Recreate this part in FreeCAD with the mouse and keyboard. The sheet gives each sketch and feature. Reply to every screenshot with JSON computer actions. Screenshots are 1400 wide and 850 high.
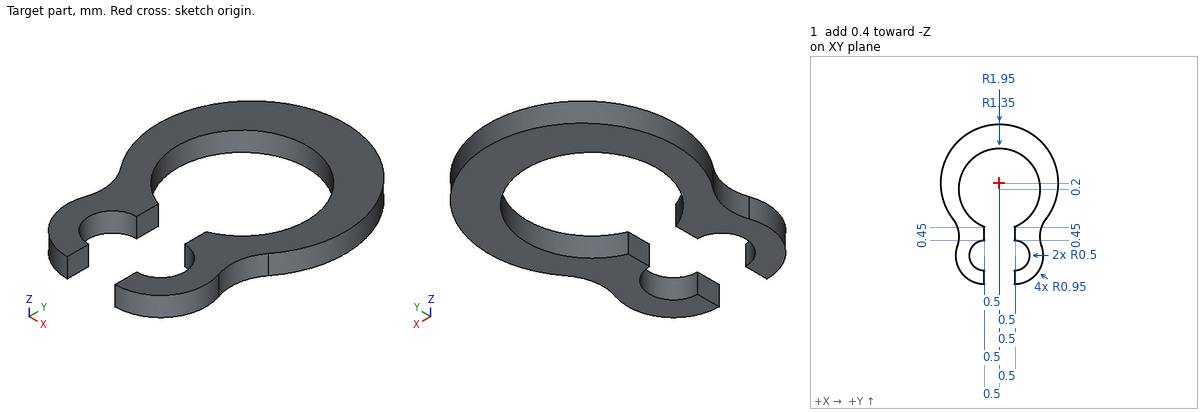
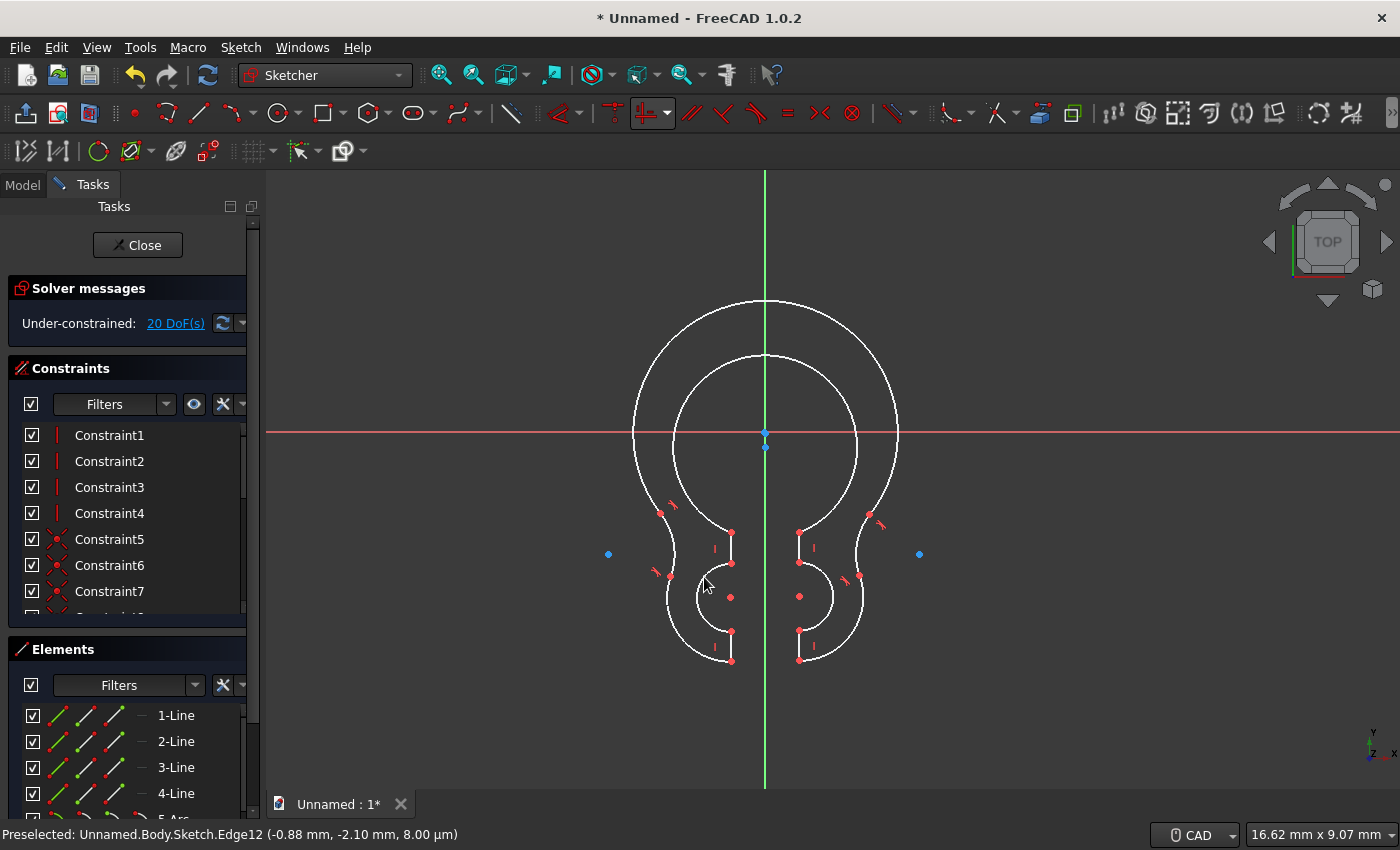
{"action": "left_click_drag", "start_coordinate": [755, 422], "coordinate": [776, 443]}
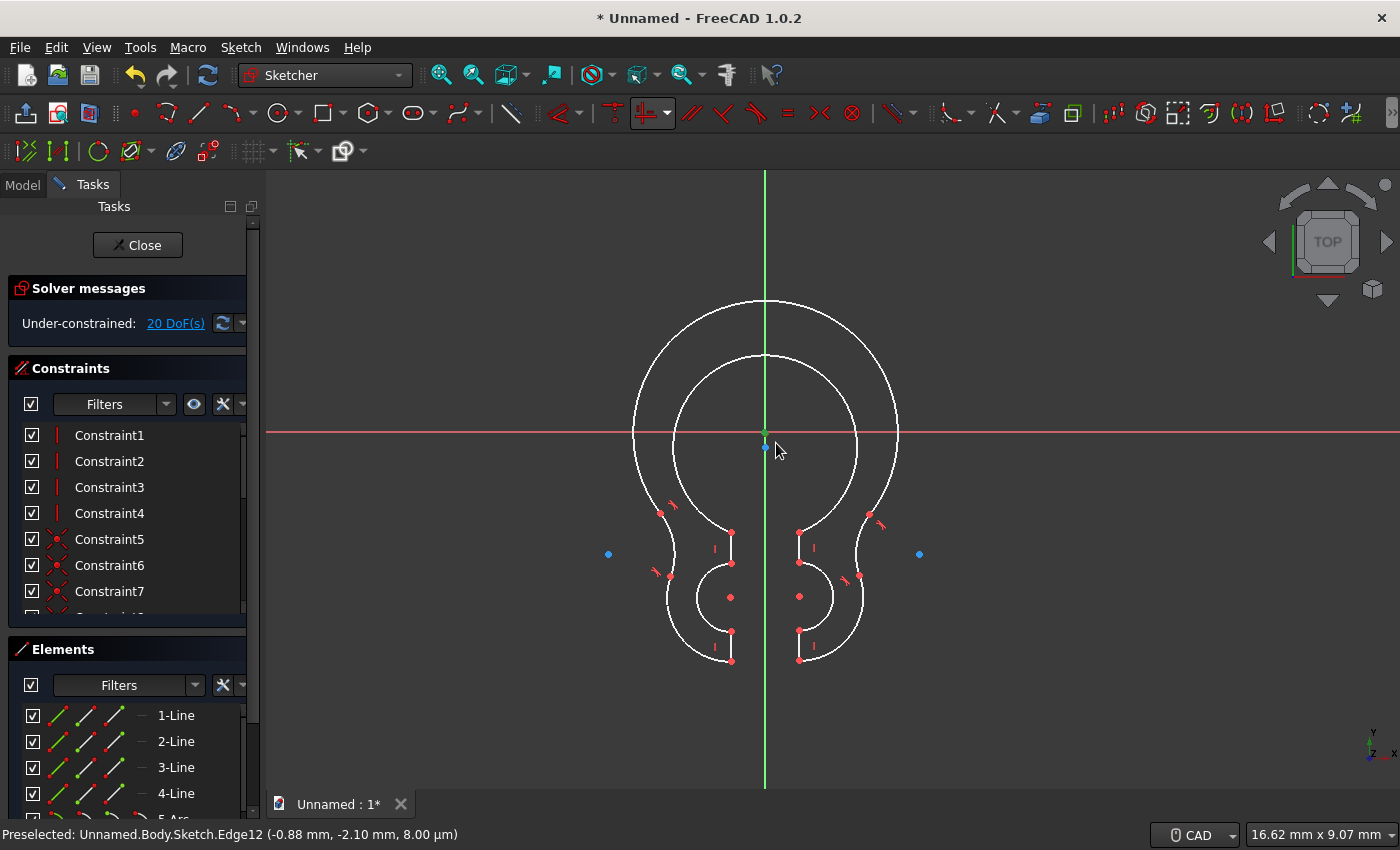
{"action": "key", "text": "c"}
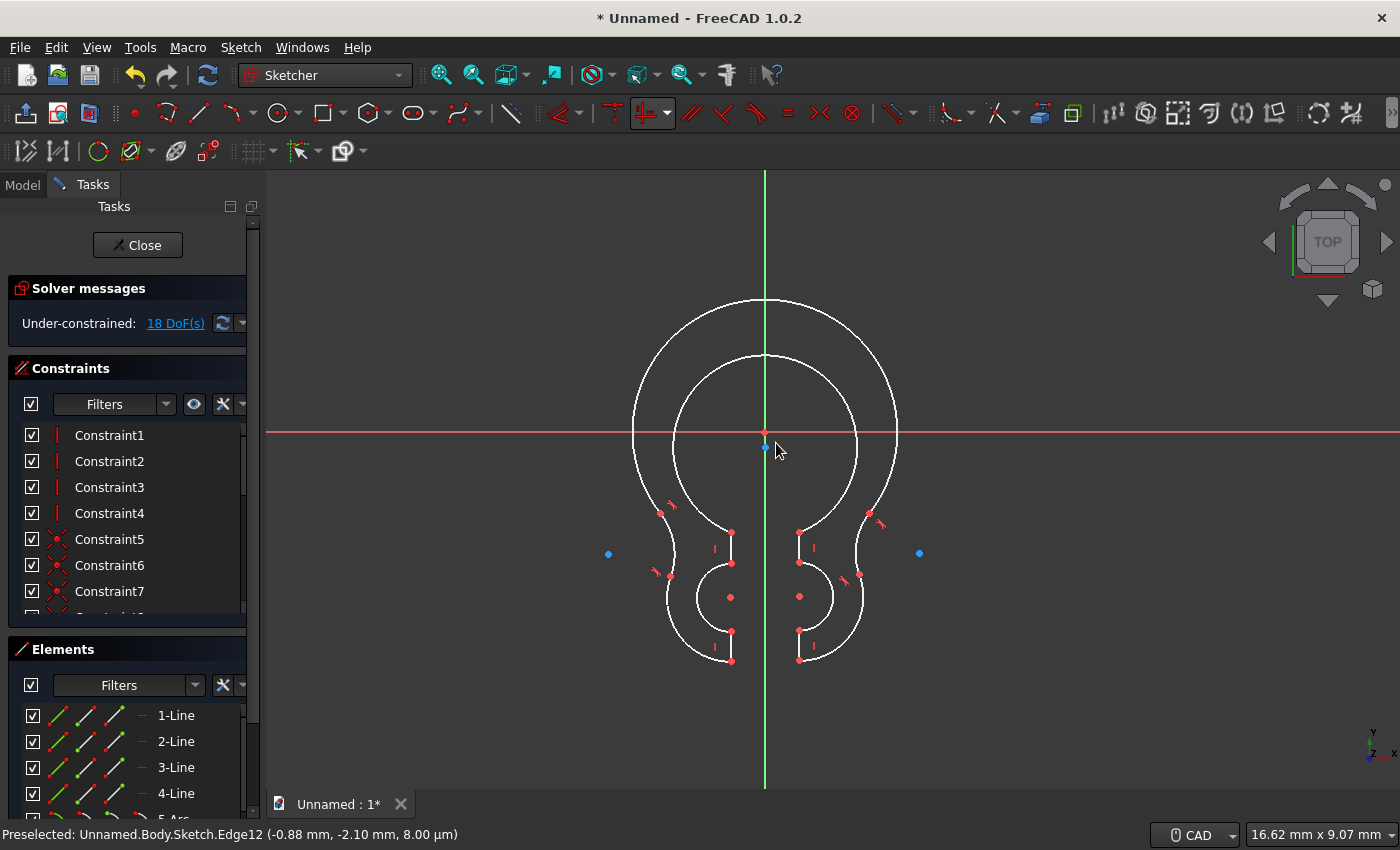
{"action": "left_click", "coordinate": [834, 651]}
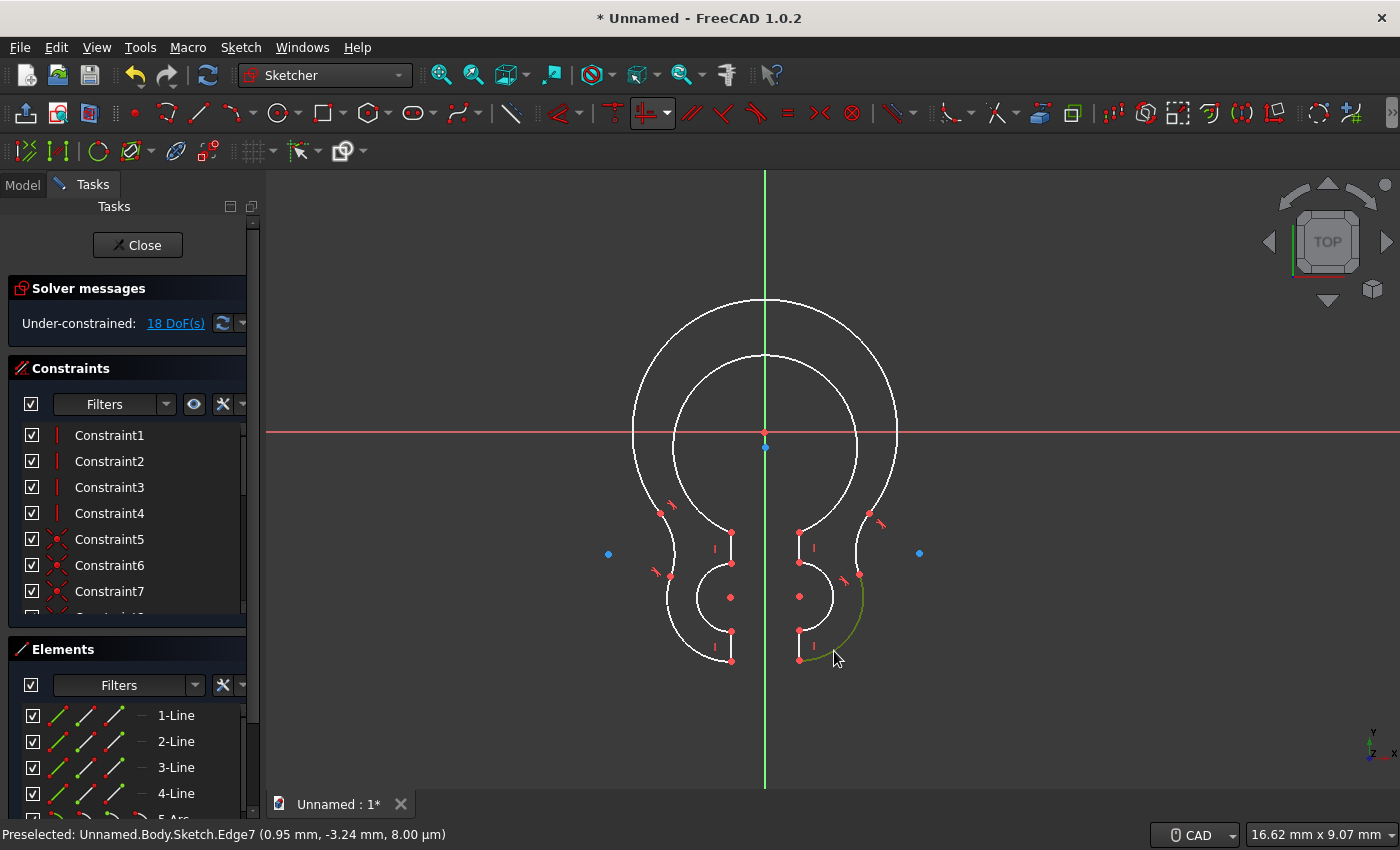
{"action": "left_click", "coordinate": [860, 531]}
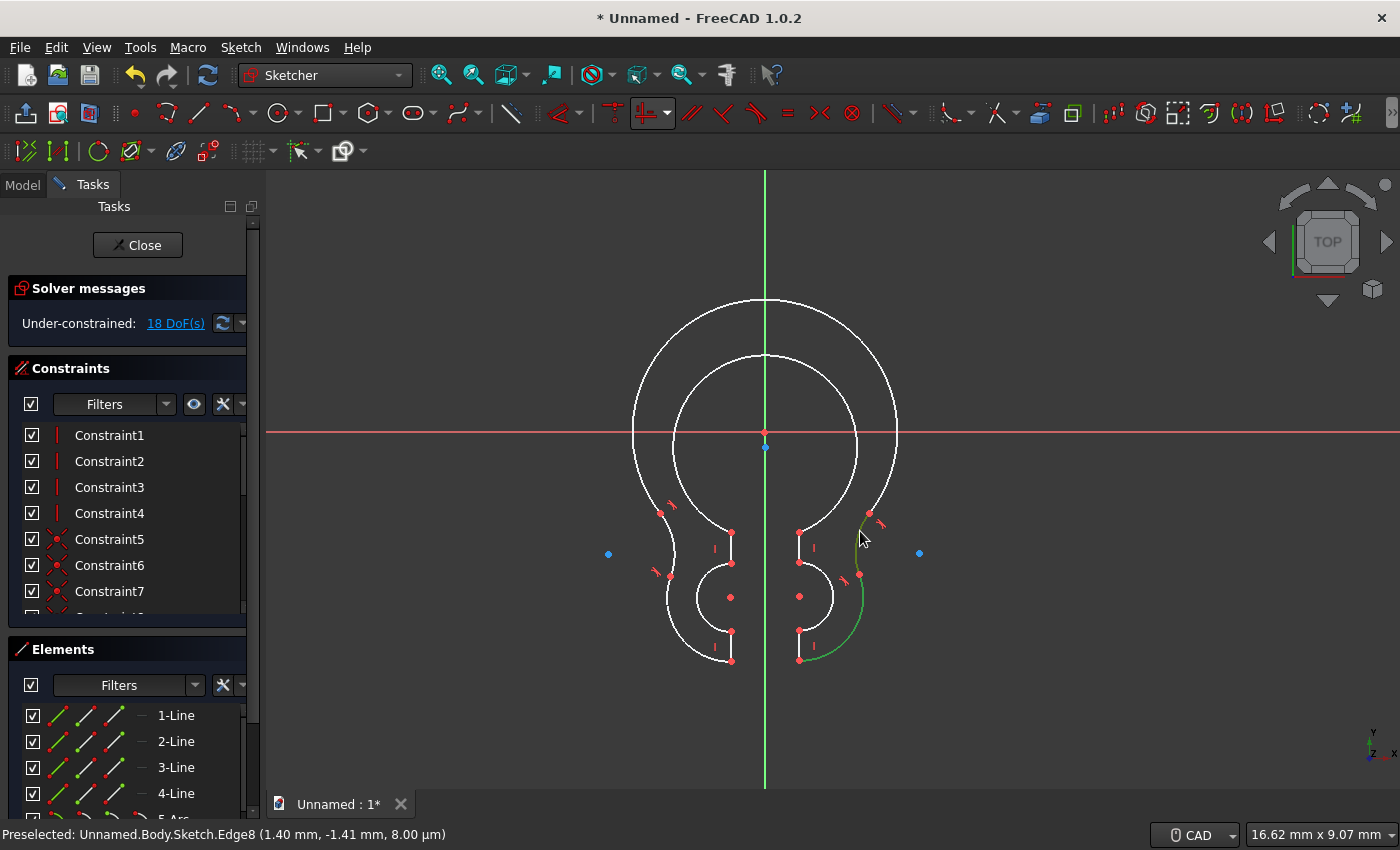
{"action": "left_click", "coordinate": [675, 557]}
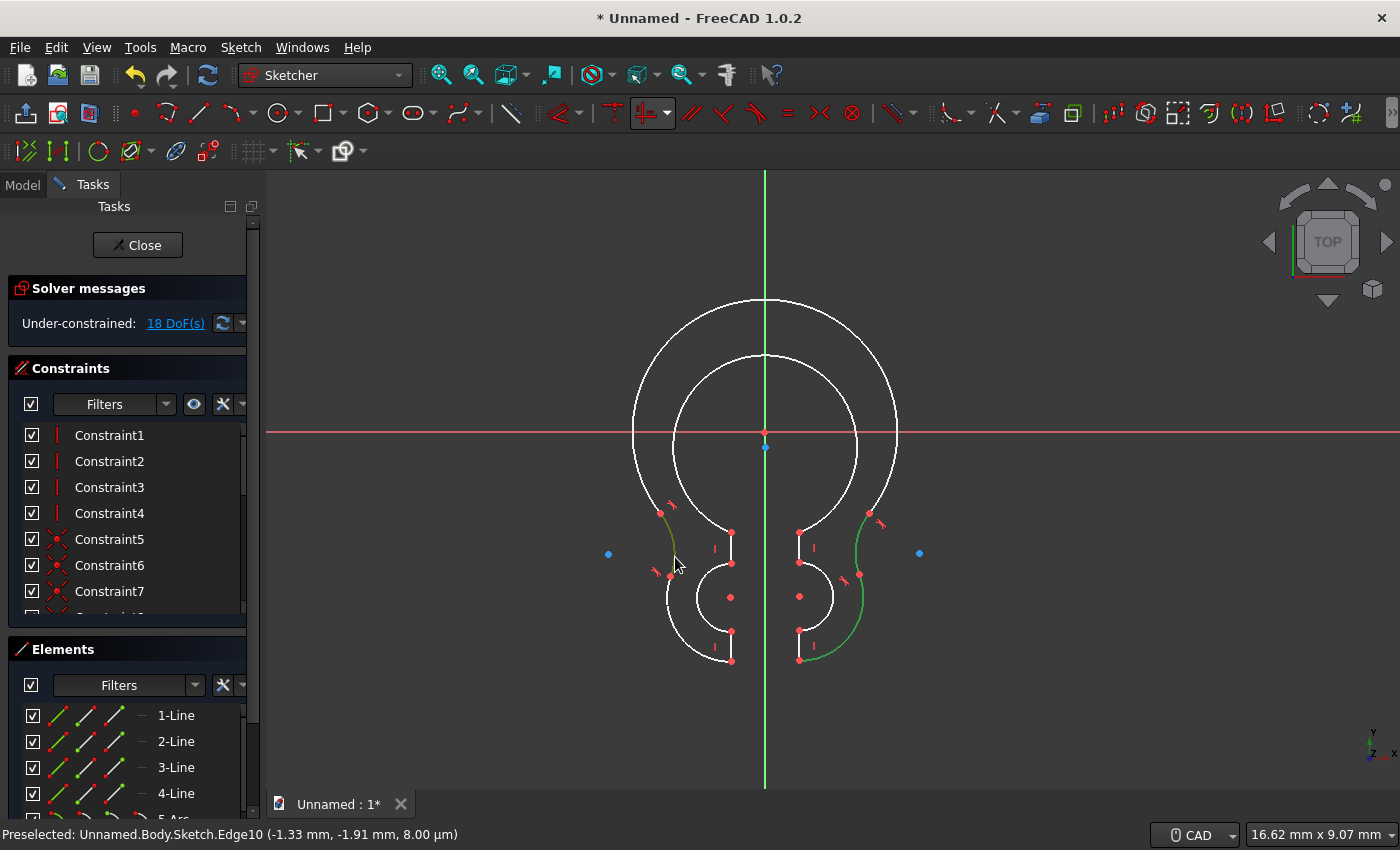
{"action": "left_click", "coordinate": [669, 613]}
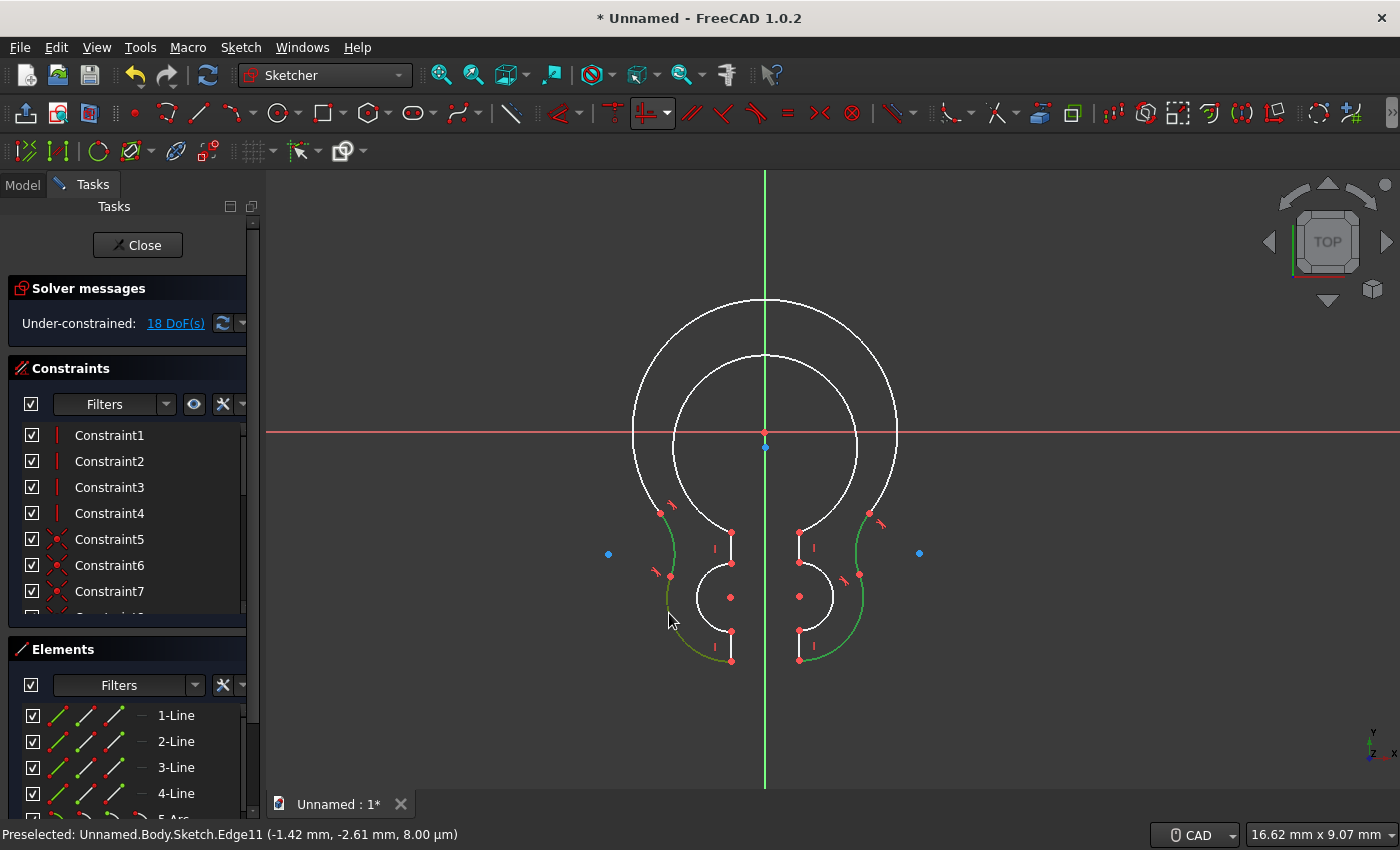
{"action": "left_click", "coordinate": [788, 114]}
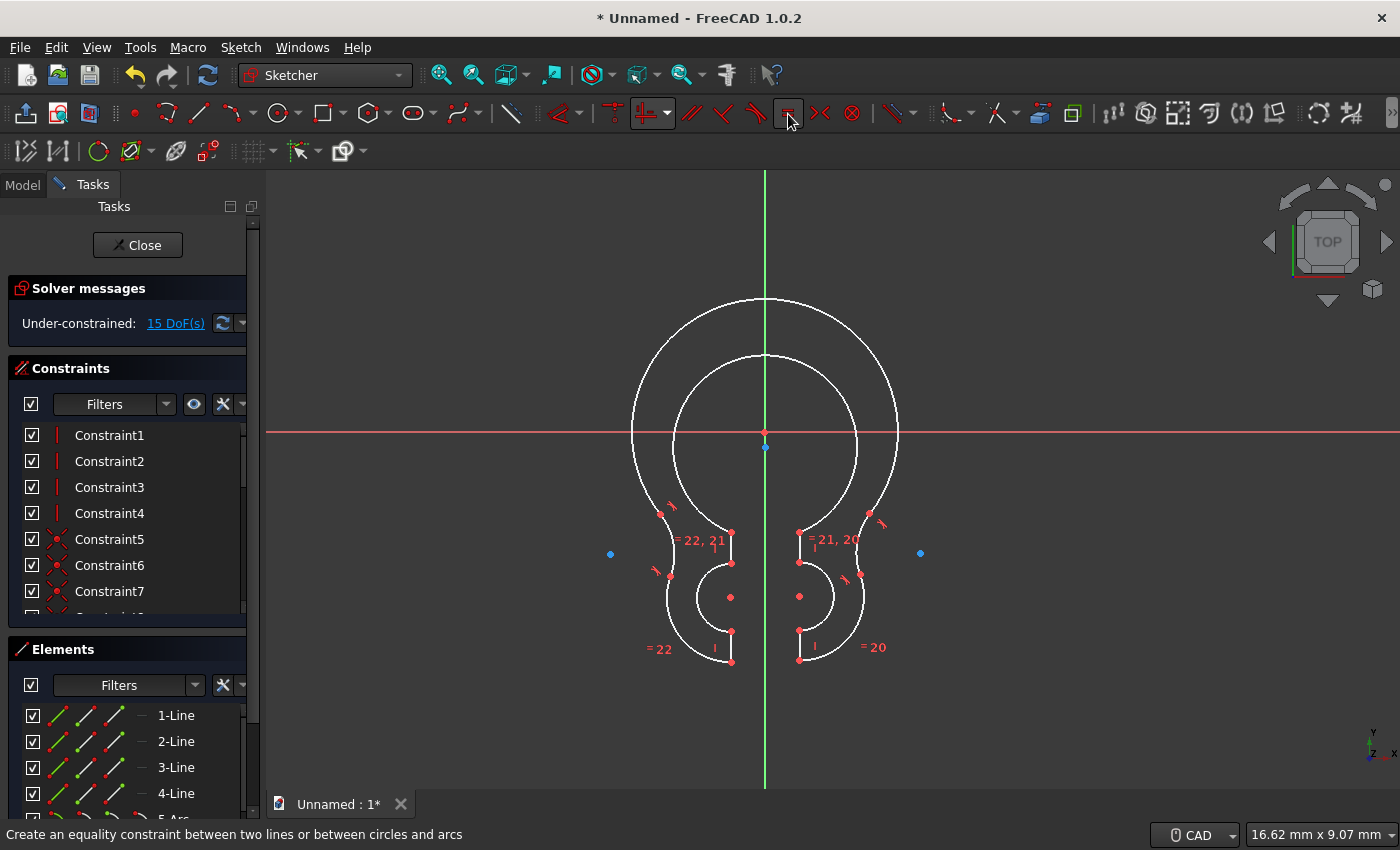
{"action": "left_click", "coordinate": [827, 616]}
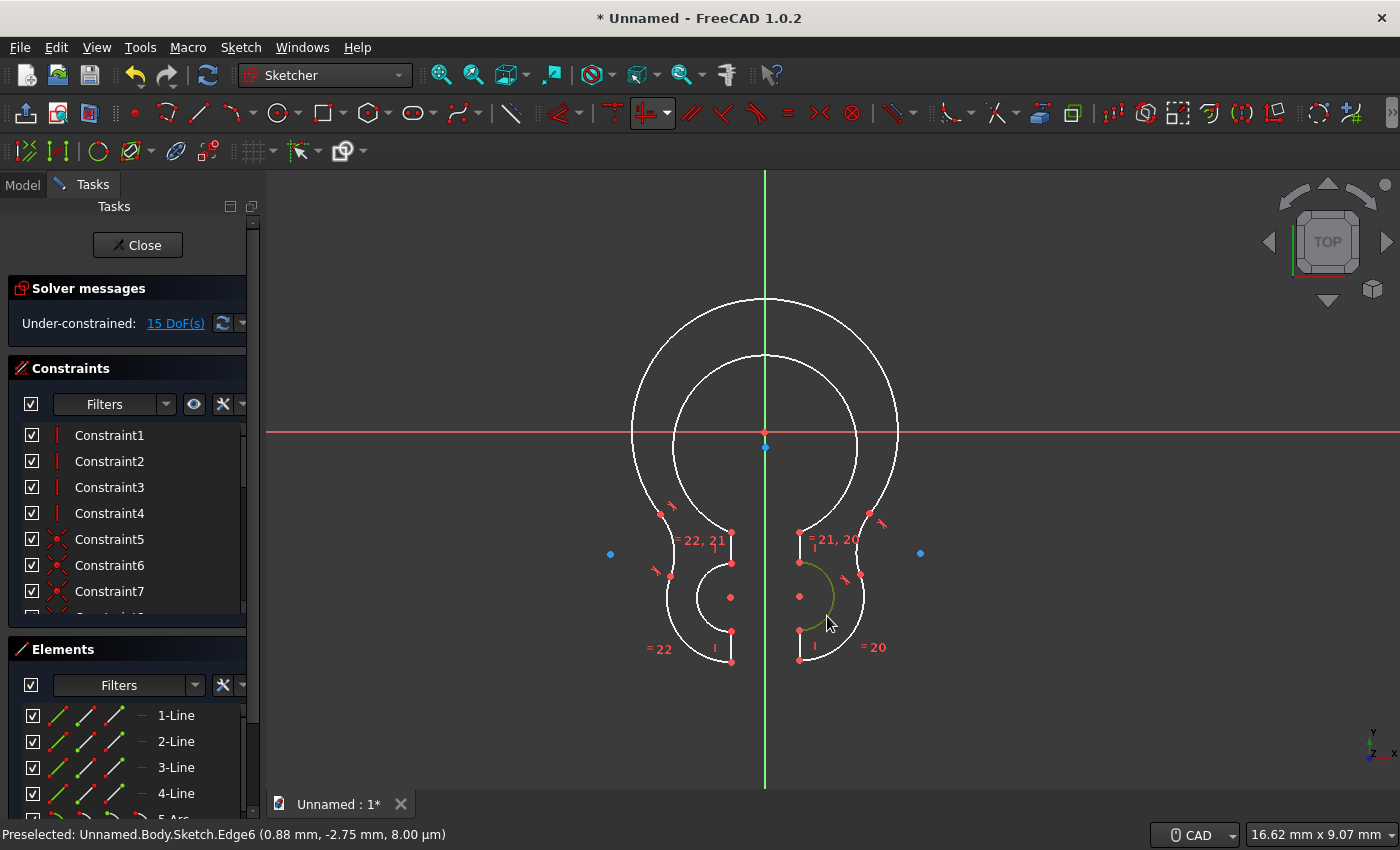
{"action": "left_click", "coordinate": [704, 578]}